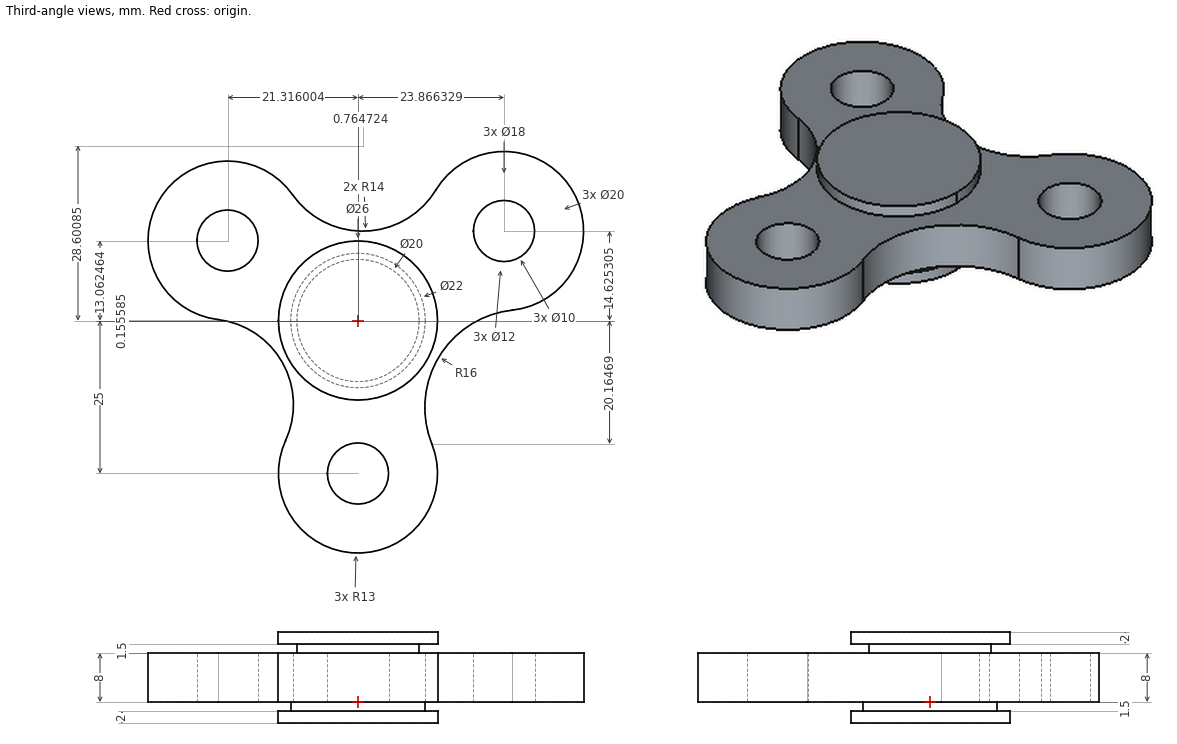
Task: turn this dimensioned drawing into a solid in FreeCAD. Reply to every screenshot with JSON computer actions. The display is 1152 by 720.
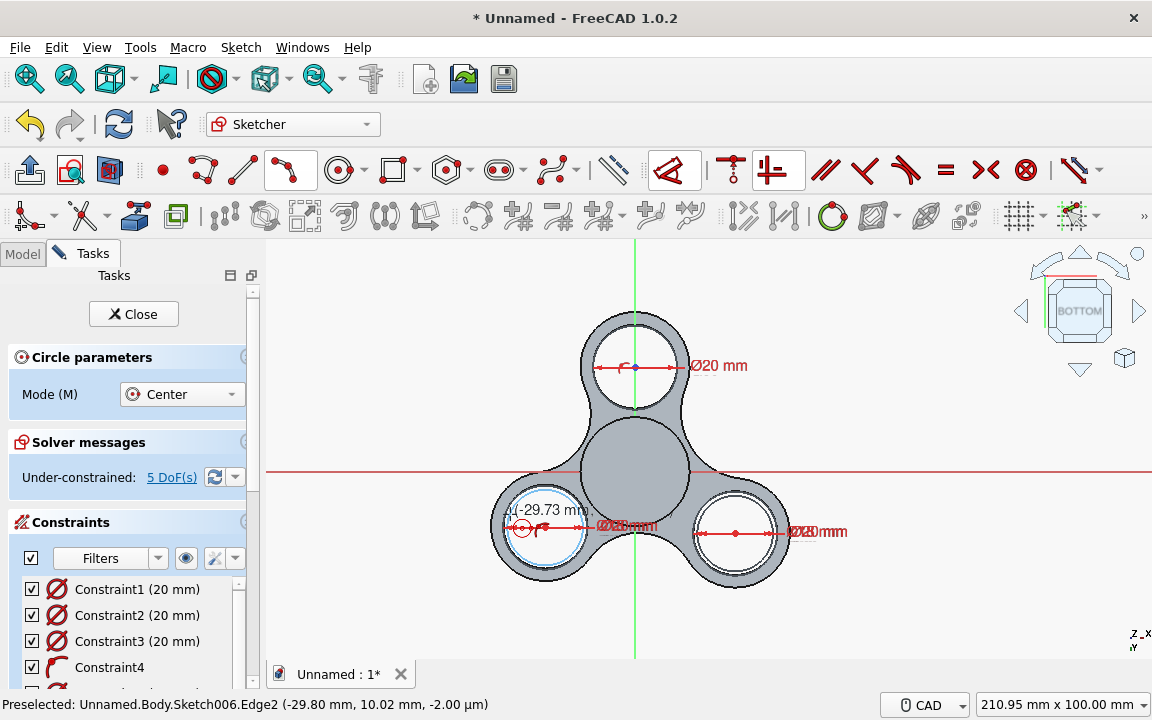
{"action": "left_click", "coordinate": [635, 368]}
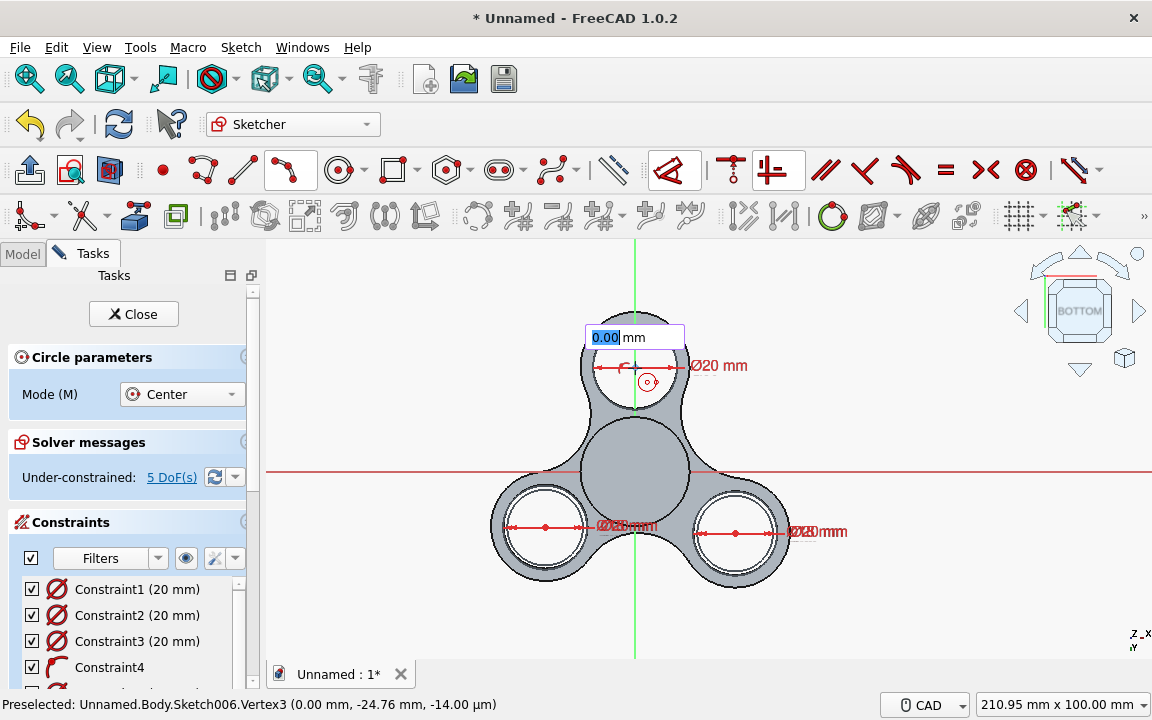
{"action": "scroll", "coordinate": [662, 393], "scroll_direction": "up", "scroll_amount": 7}
{"action": "mouse_move", "coordinate": [660, 393]}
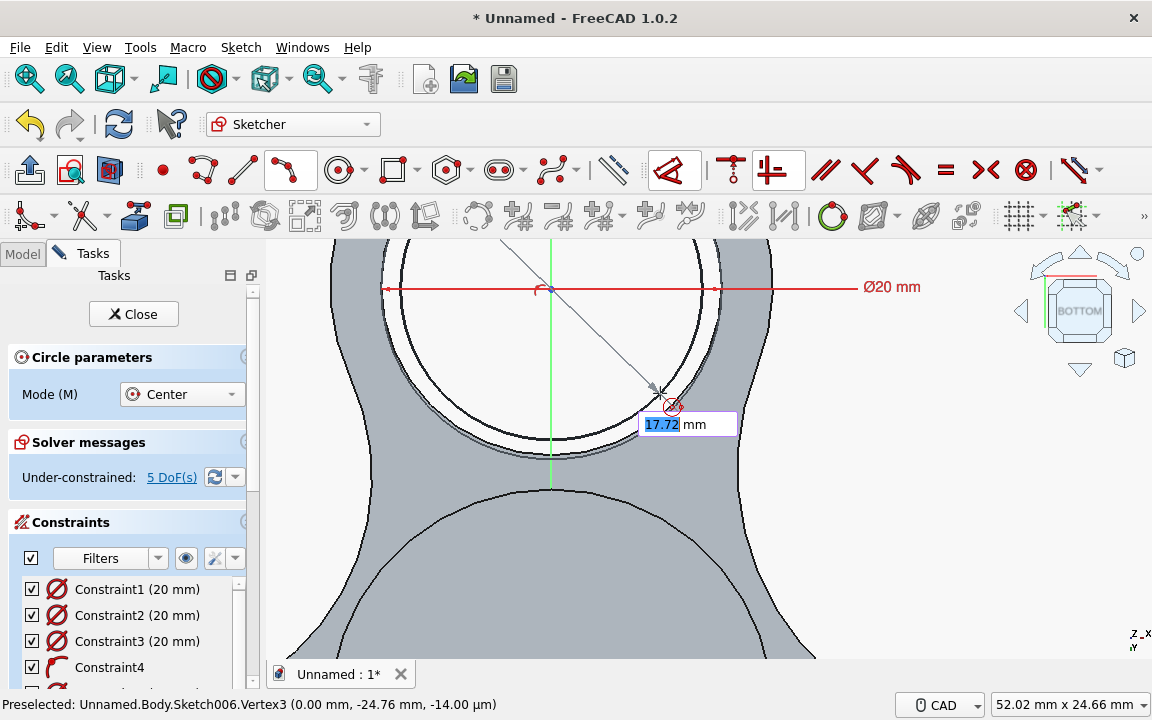
{"action": "type", "text": "18"}
{"action": "key", "text": "Return"}
{"action": "key", "text": "Escape"}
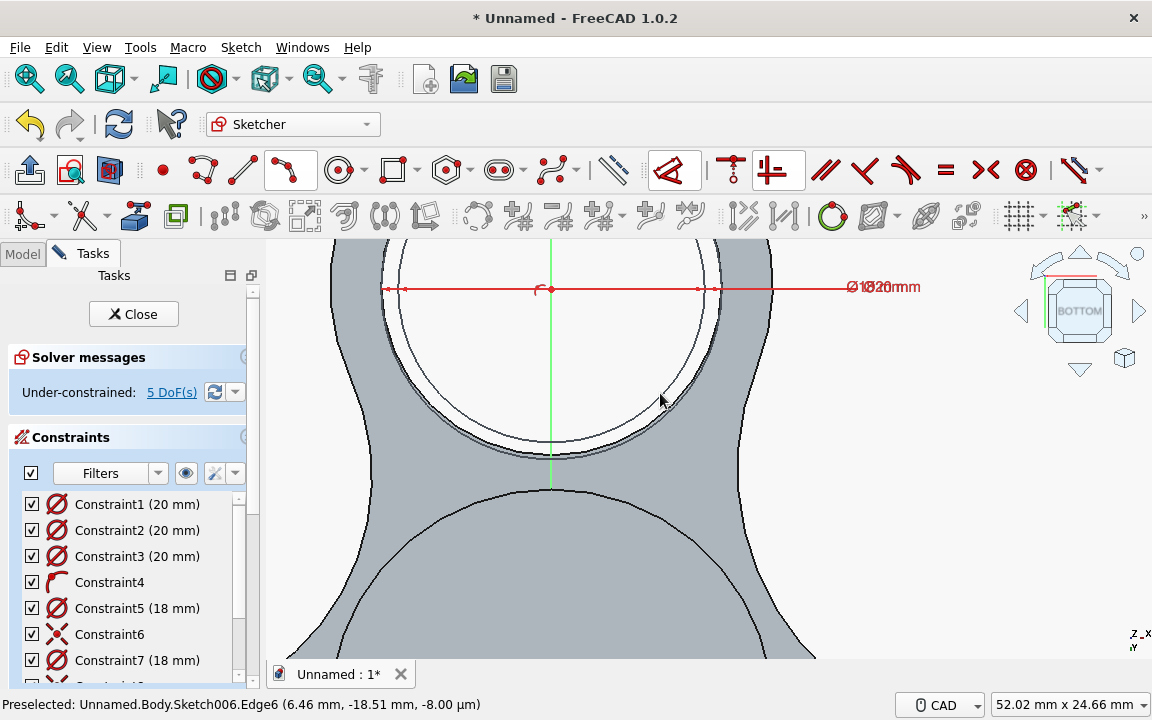
{"action": "scroll", "coordinate": [663, 392], "scroll_direction": "down", "scroll_amount": 7}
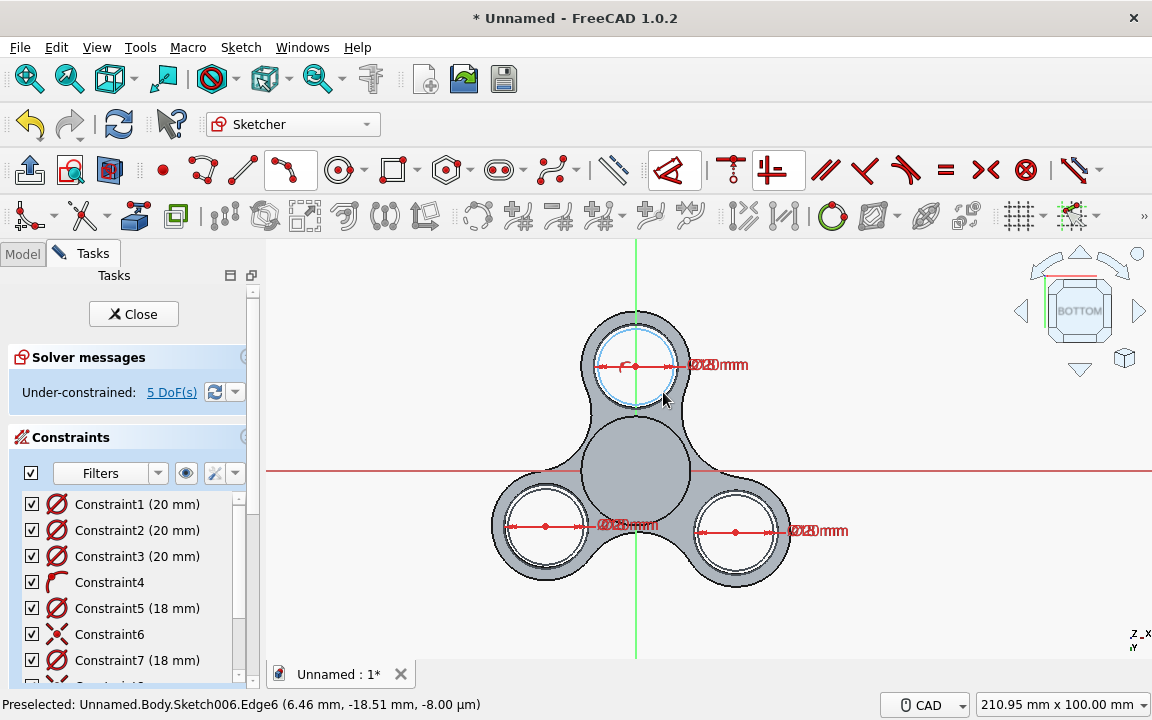
{"action": "left_click", "coordinate": [636, 367]}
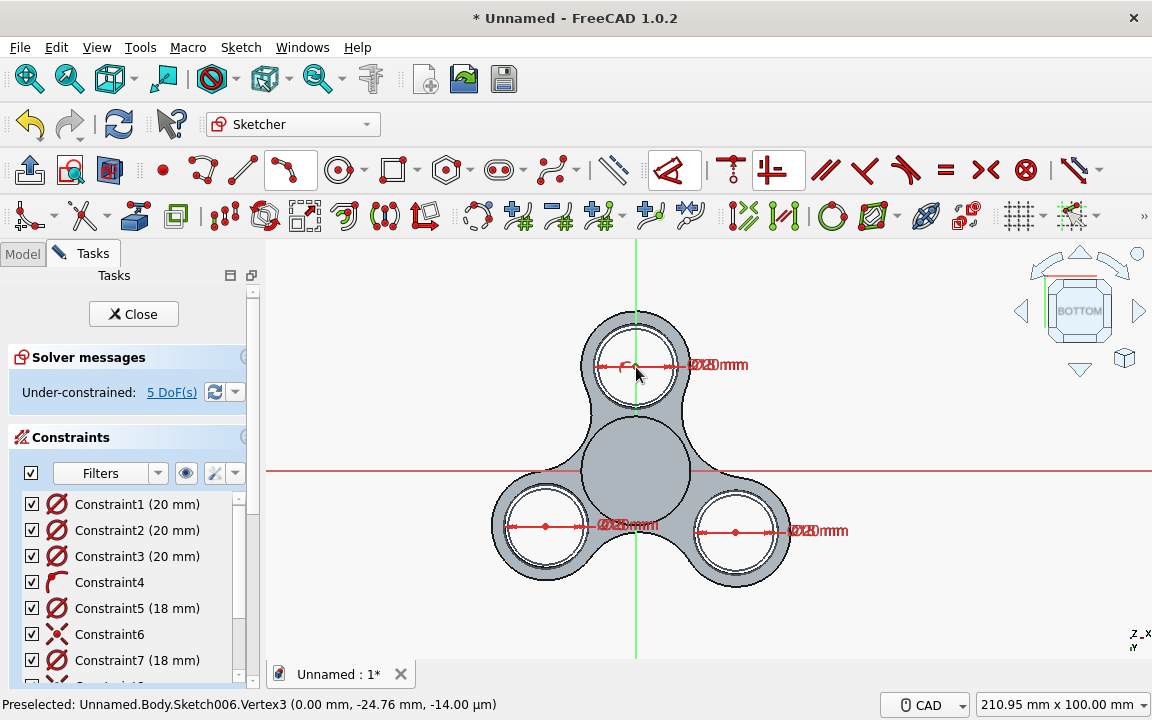
{"action": "key", "text": "i"}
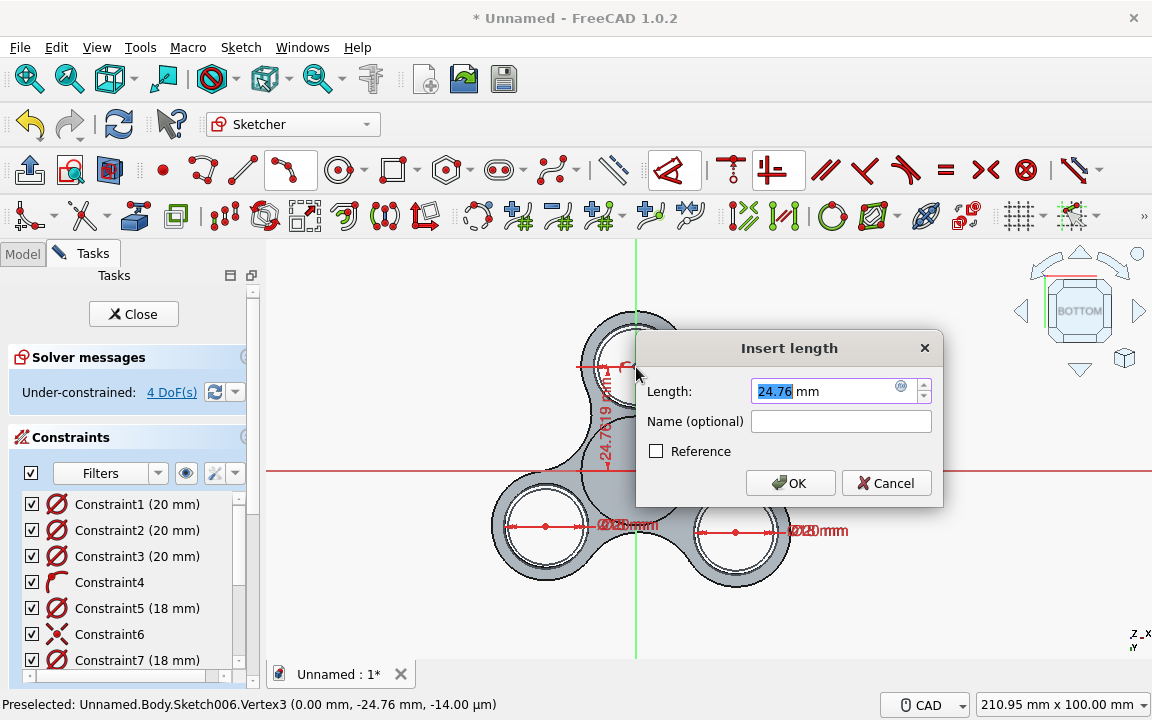
{"action": "type", "text": "25"}
{"action": "key", "text": "Return"}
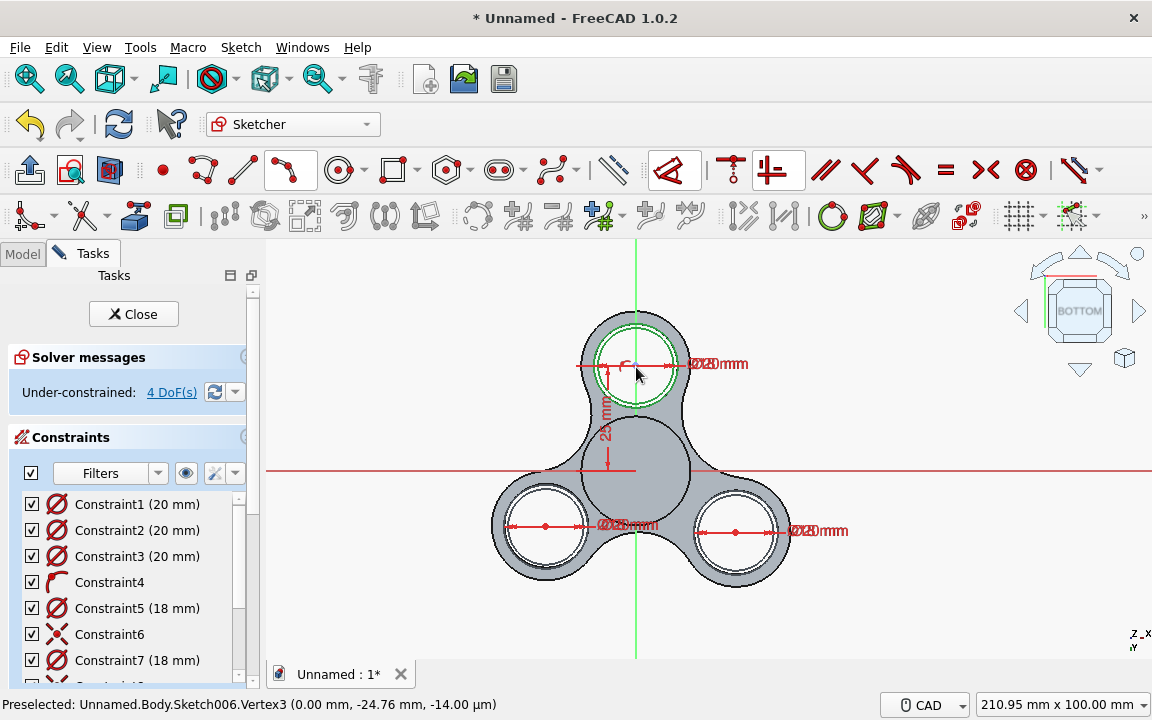
{"action": "left_click", "coordinate": [736, 533]}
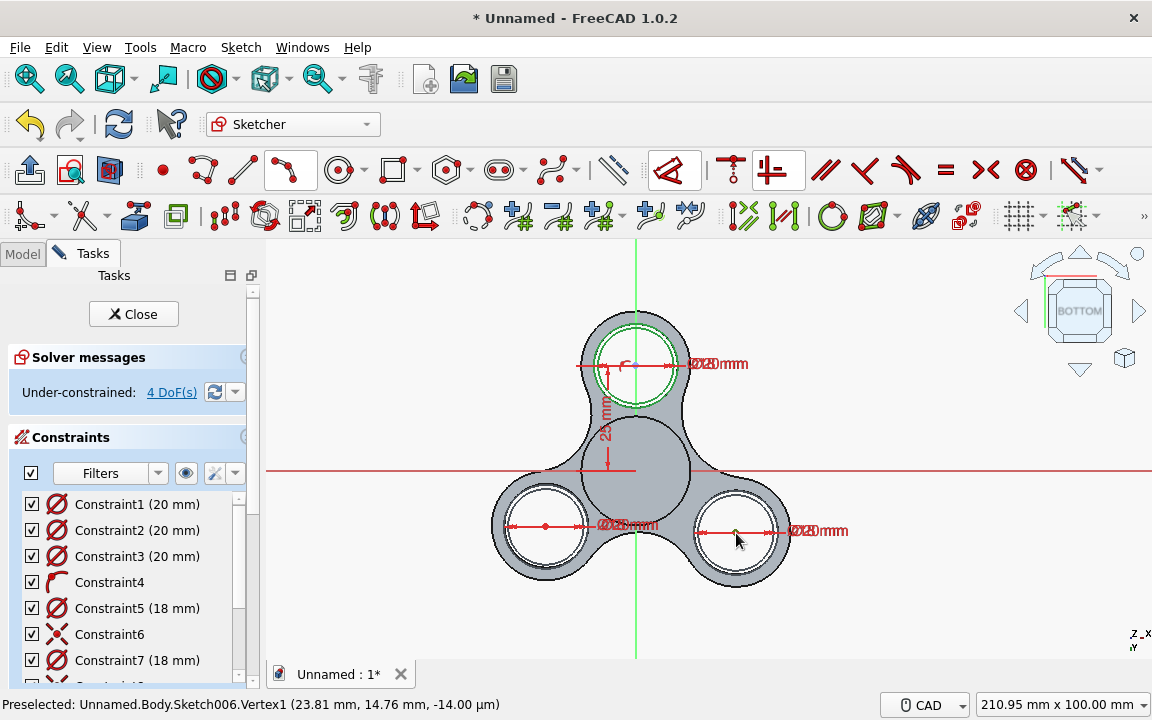
{"action": "key", "text": "l"}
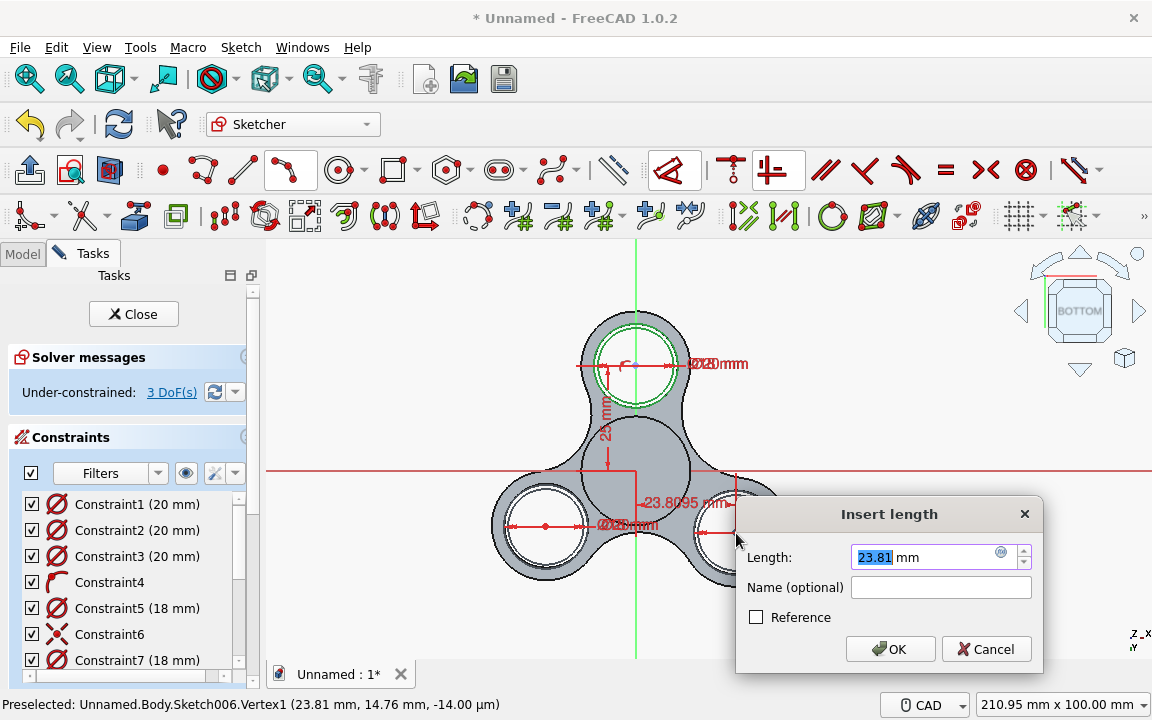
{"action": "type", "text": "23.866329"}
{"action": "key", "text": "Return"}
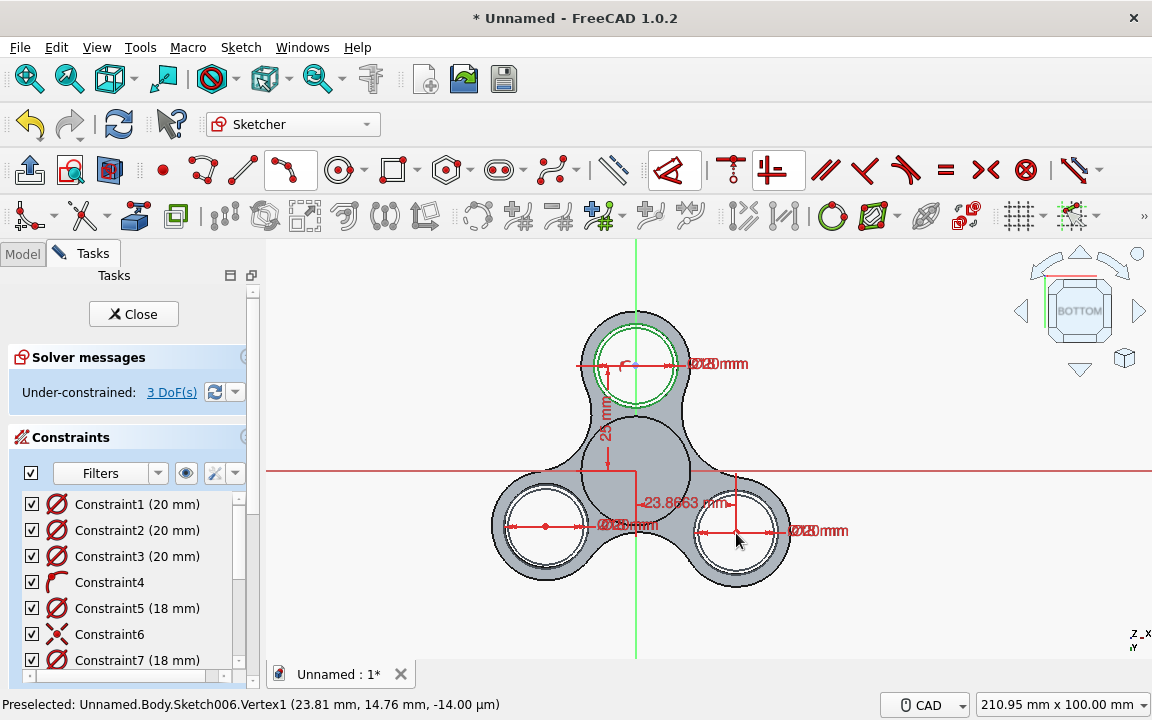
{"action": "left_click", "coordinate": [736, 533]}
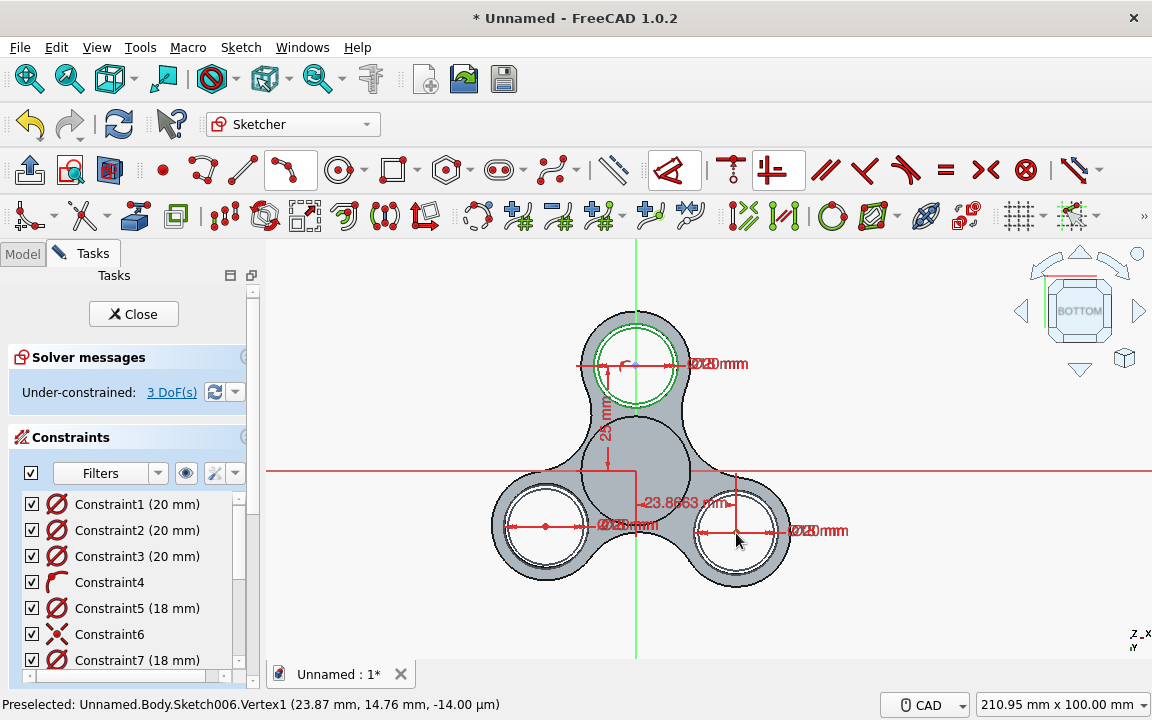
{"action": "key", "text": "i"}